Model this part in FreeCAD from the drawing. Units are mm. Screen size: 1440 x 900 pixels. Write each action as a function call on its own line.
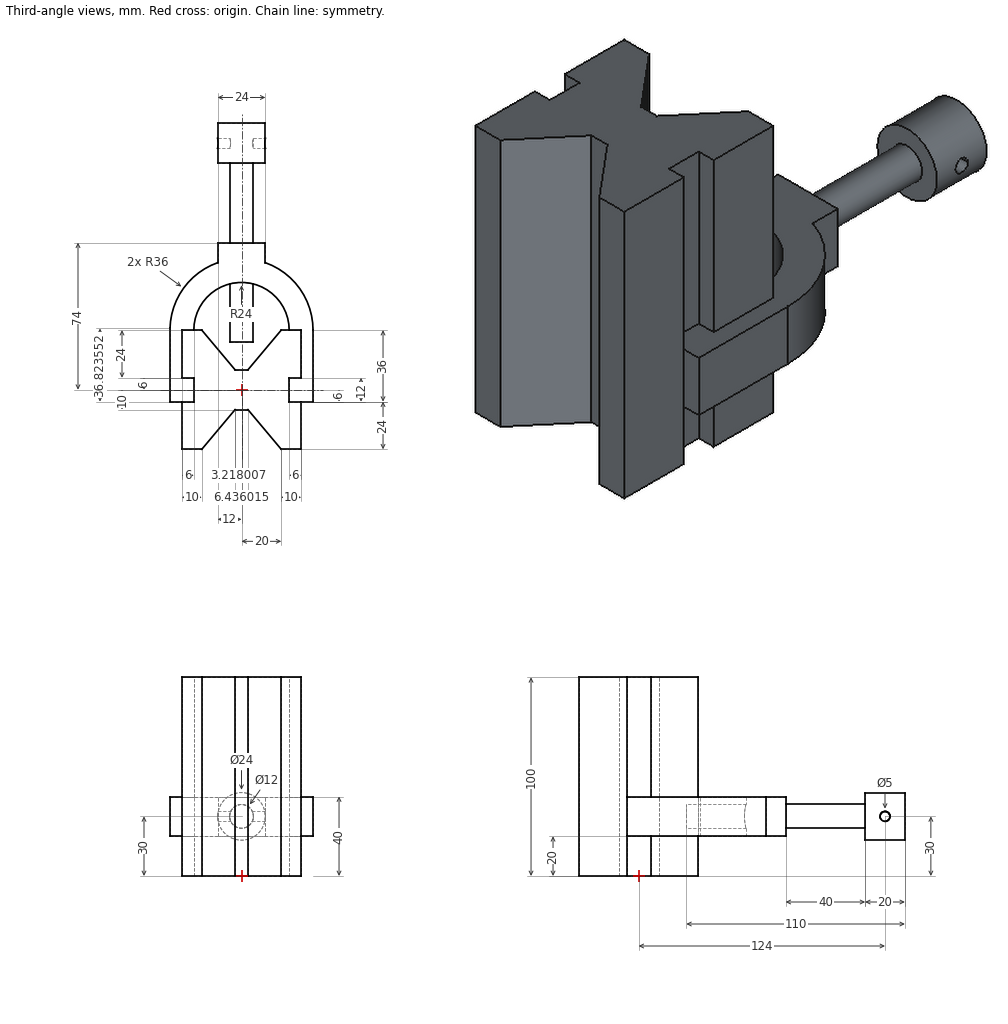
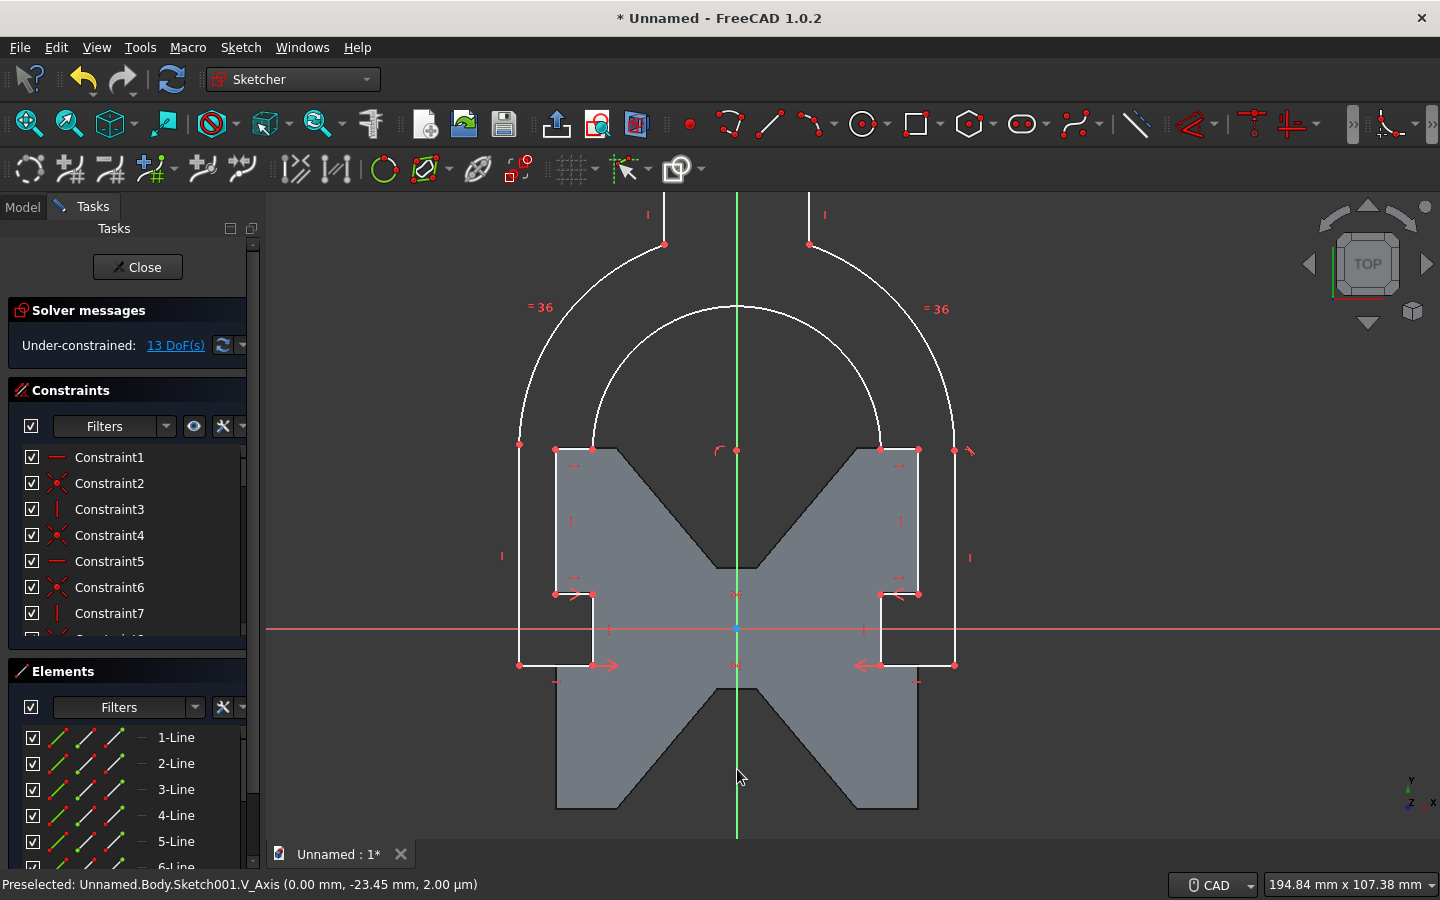
click(1190, 124)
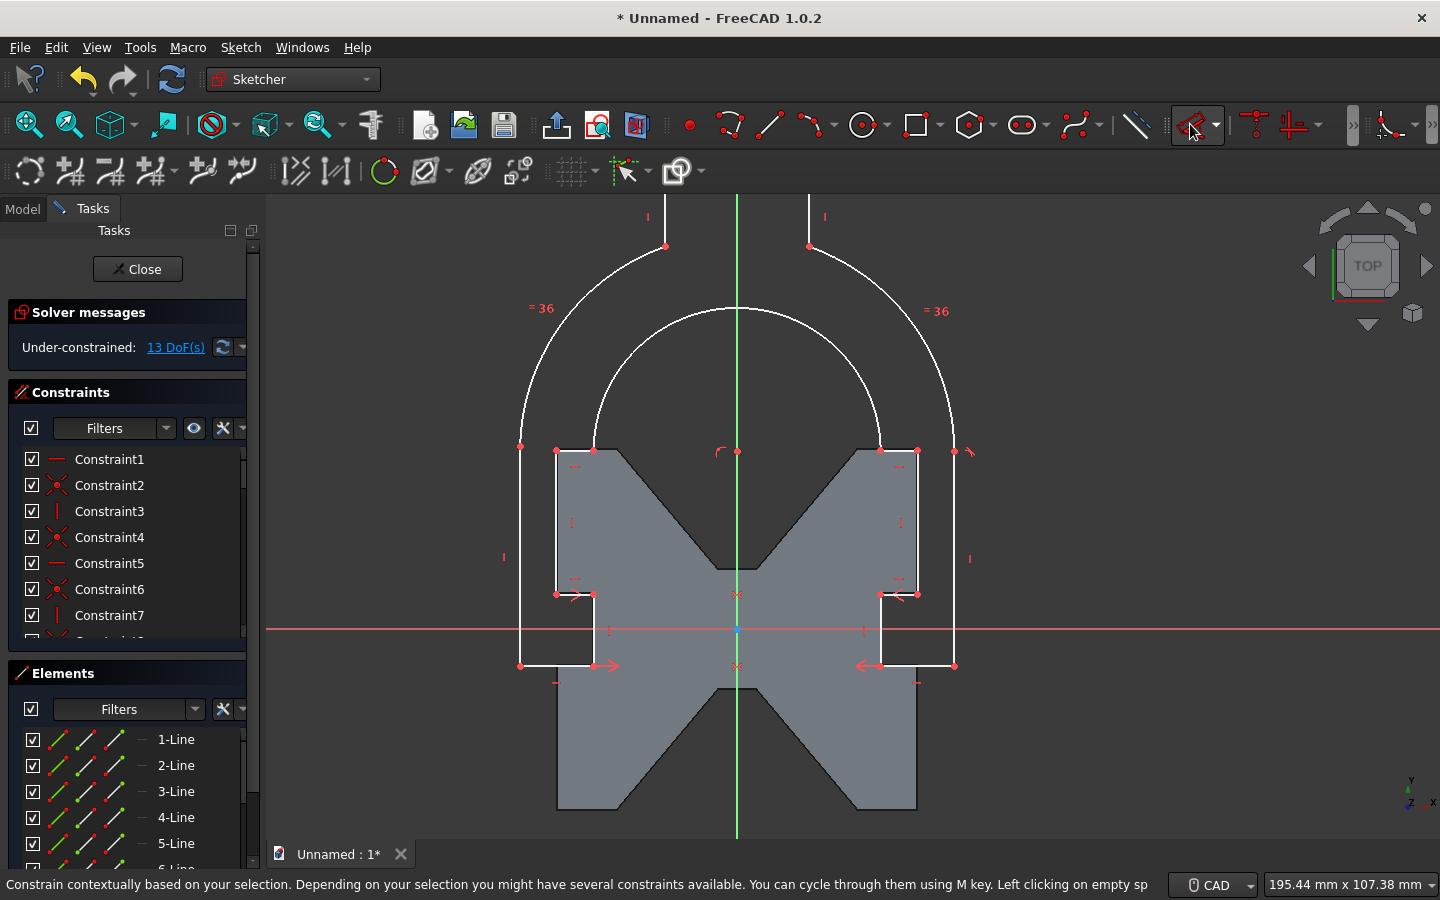
click(597, 286)
click(576, 262)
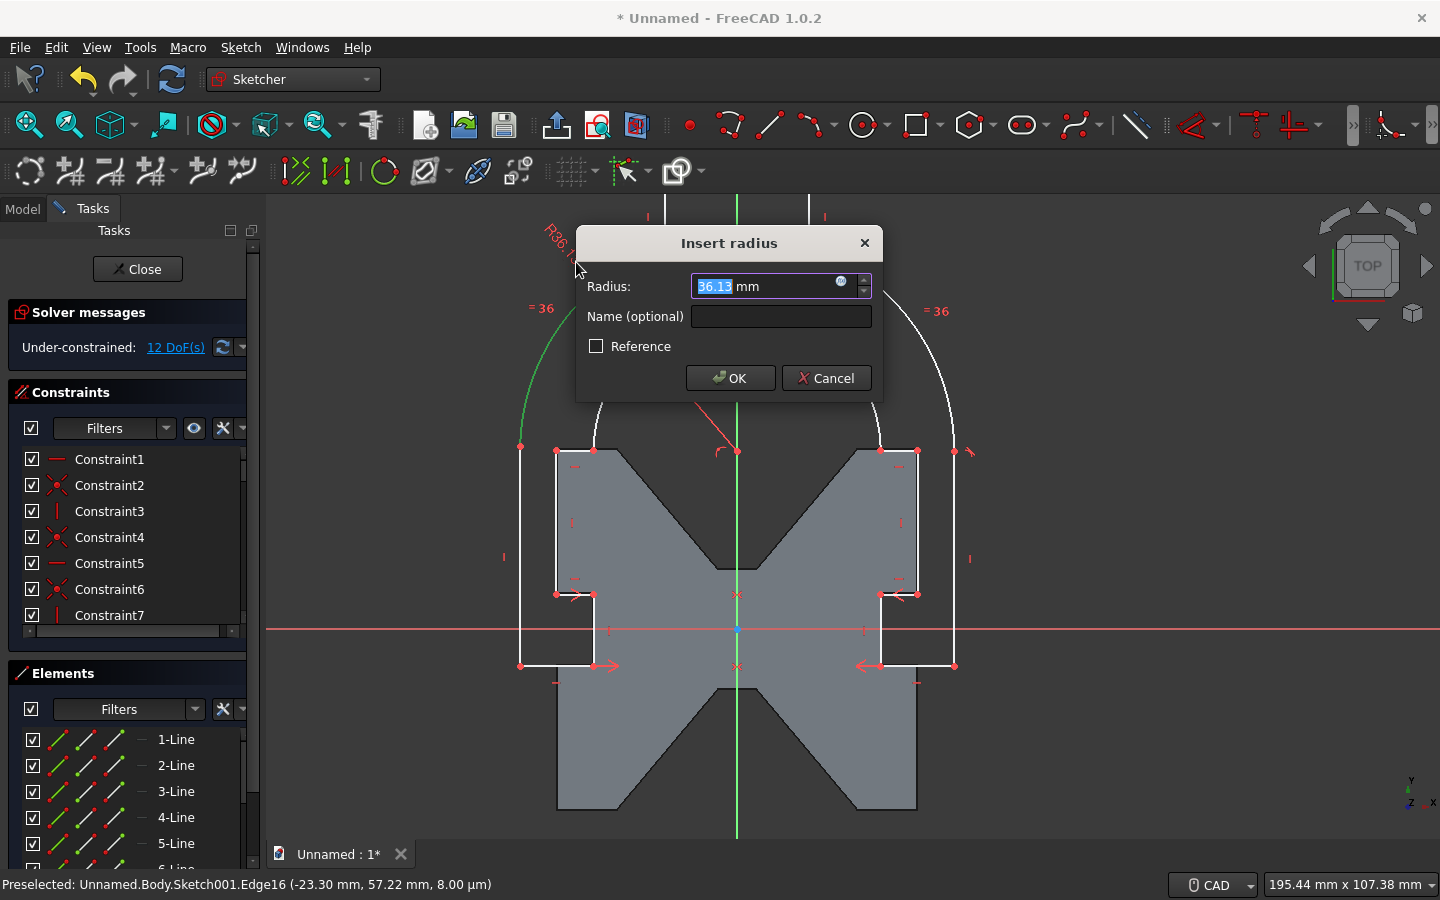
text(36)
key(Return)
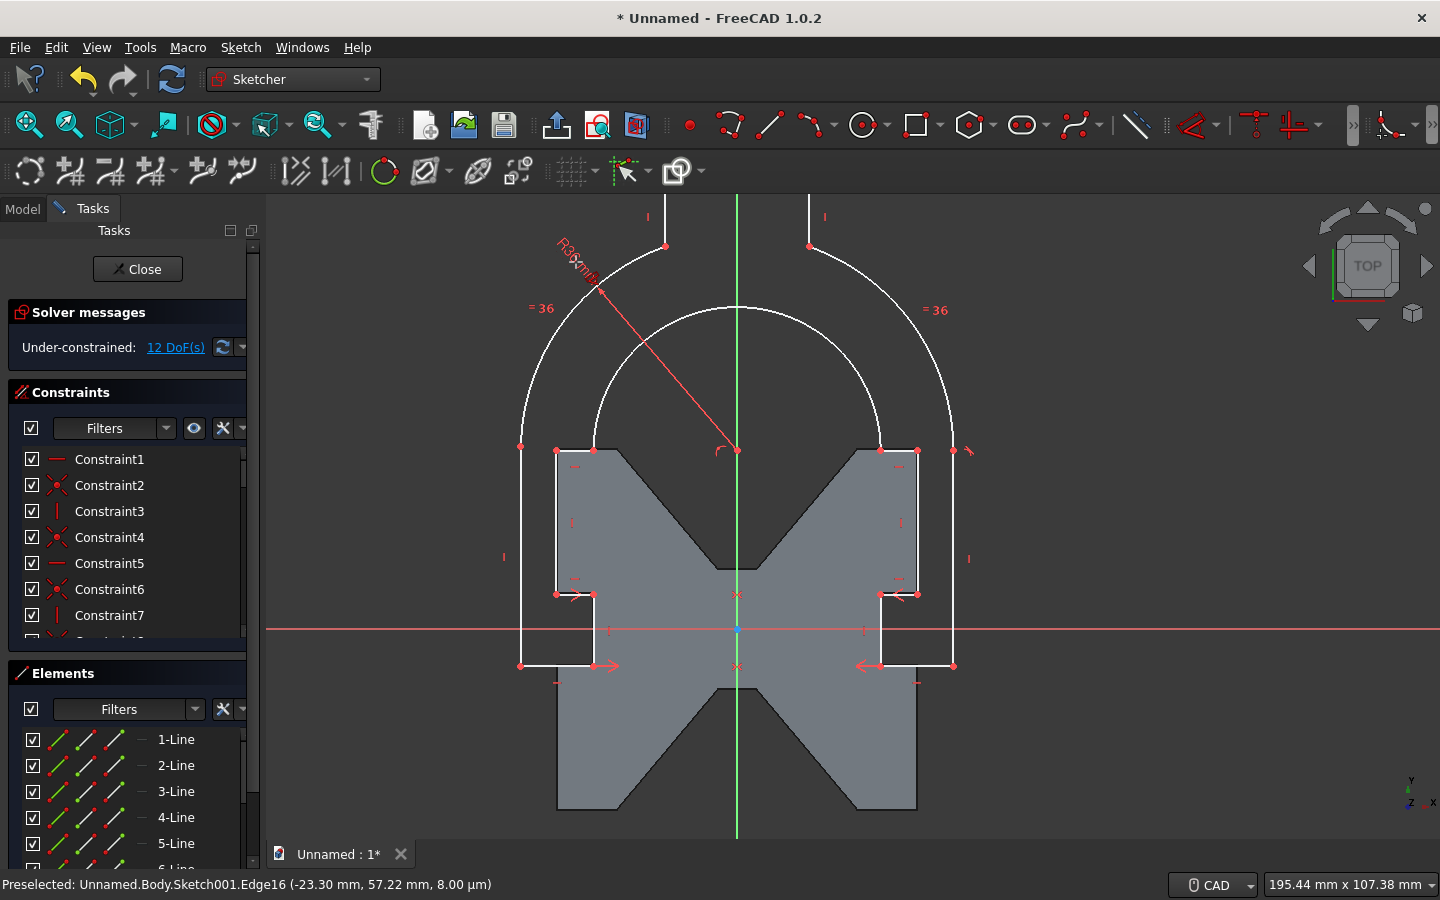
click(821, 334)
click(840, 308)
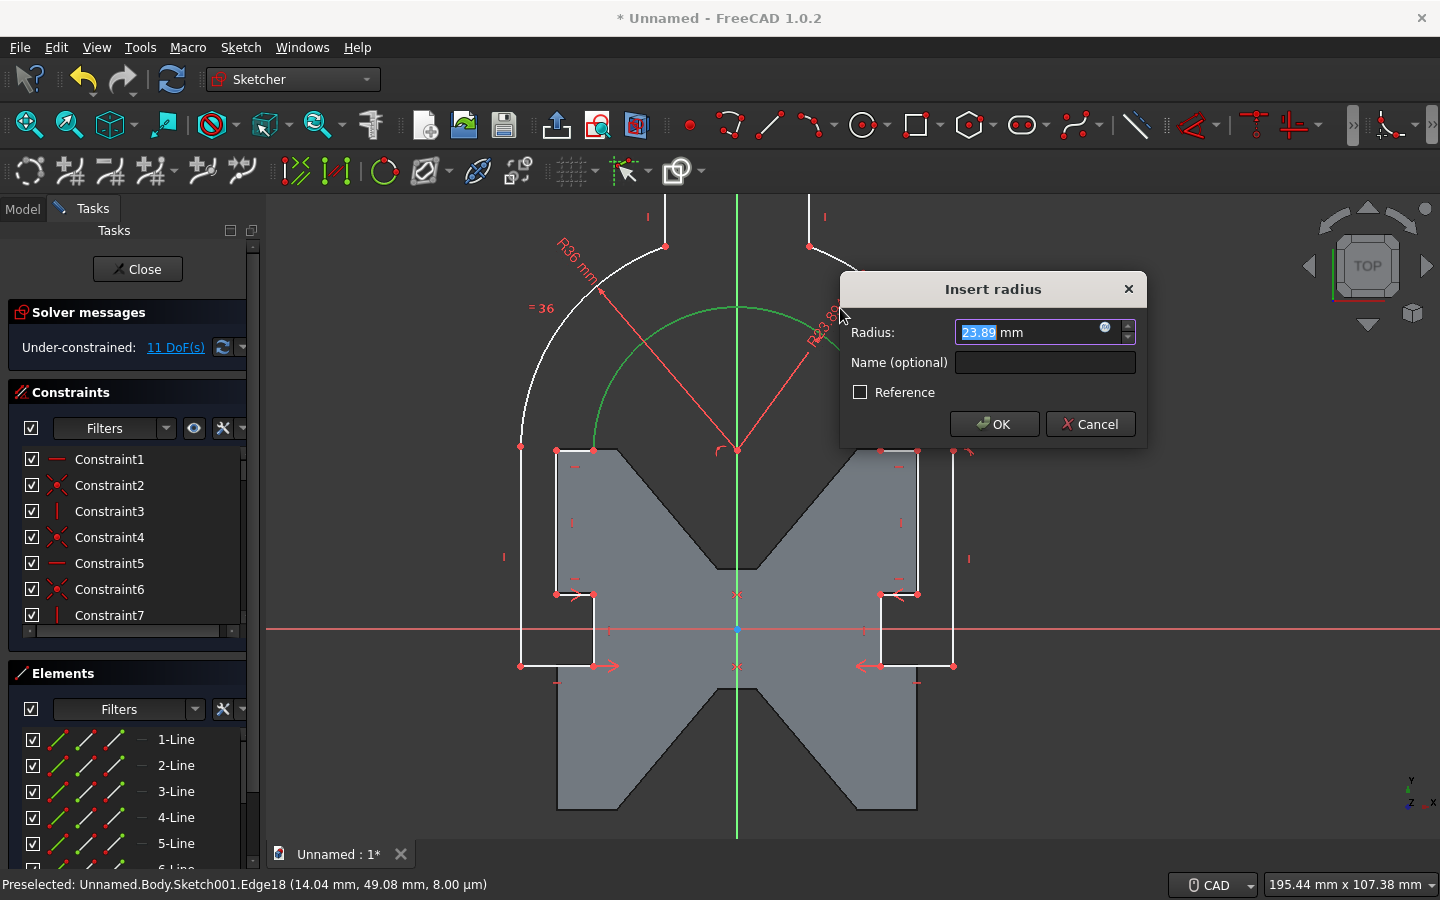
text(24)
key(Return)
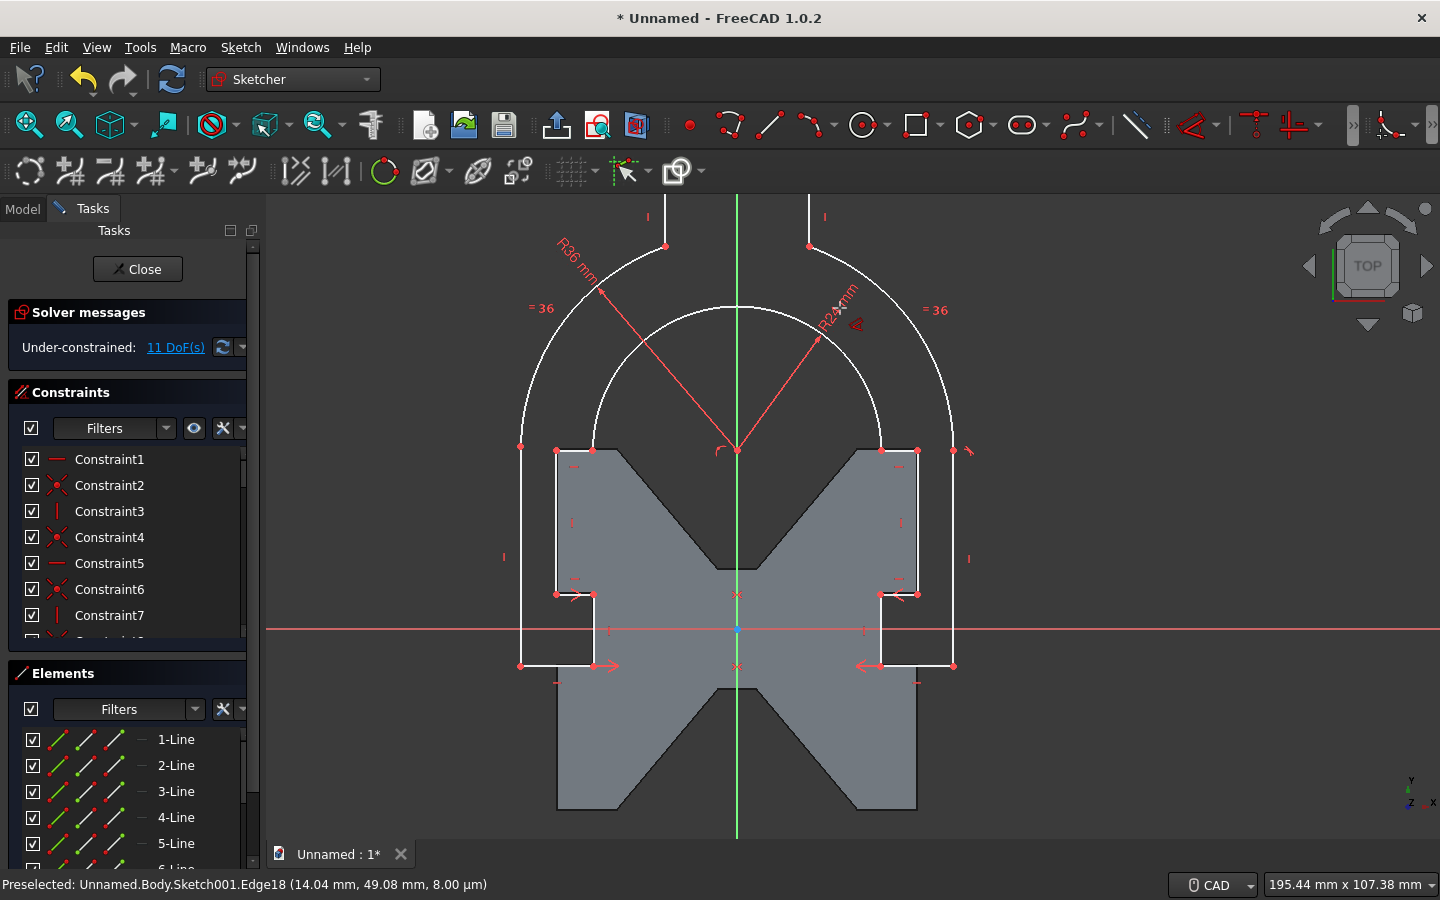
scroll(582, 451, up, 2)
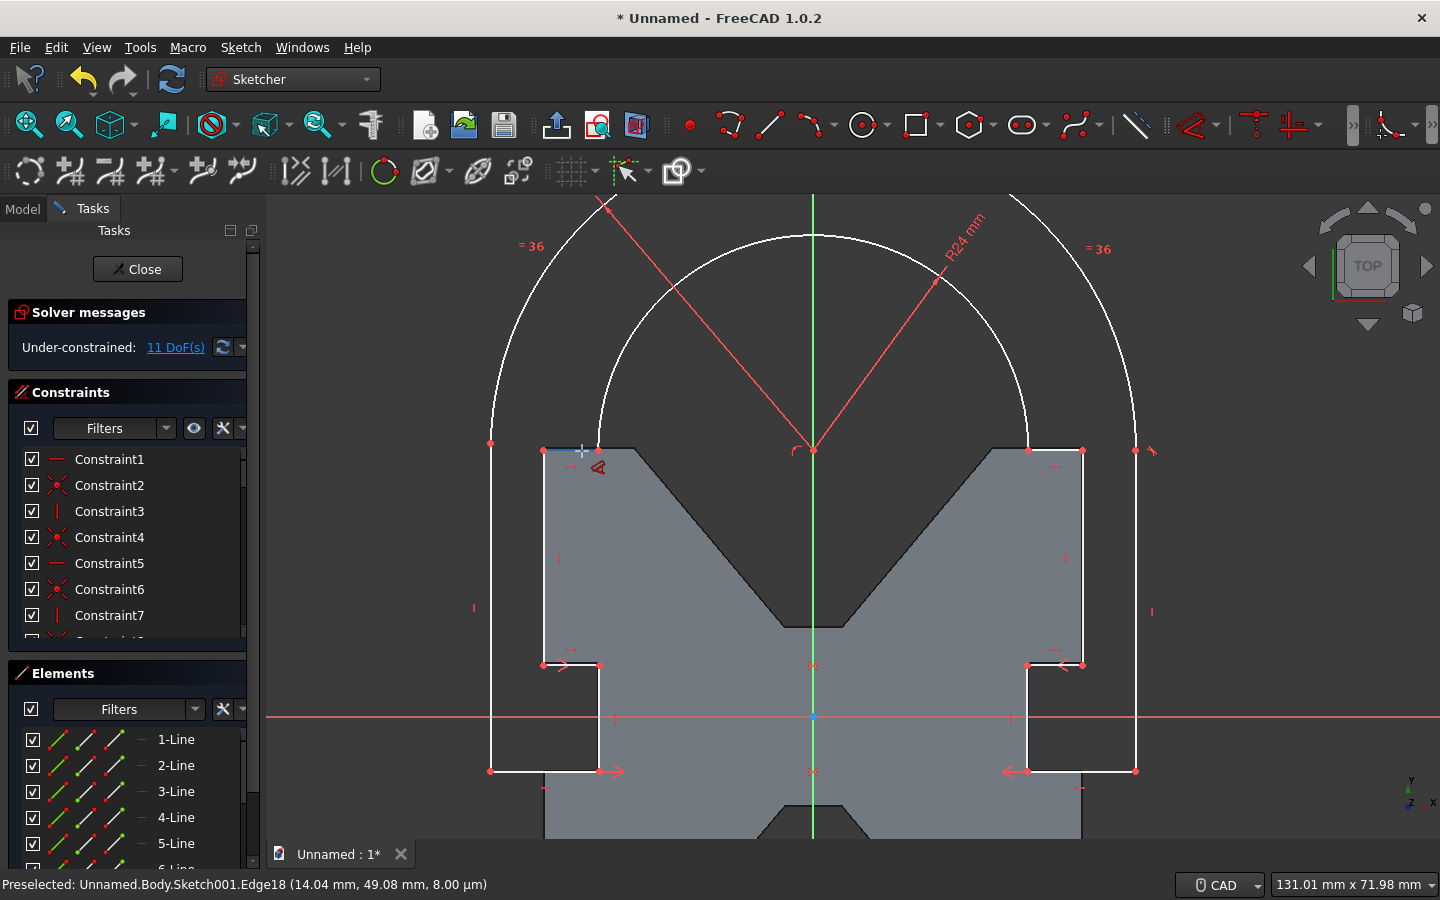
click(582, 450)
click(571, 484)